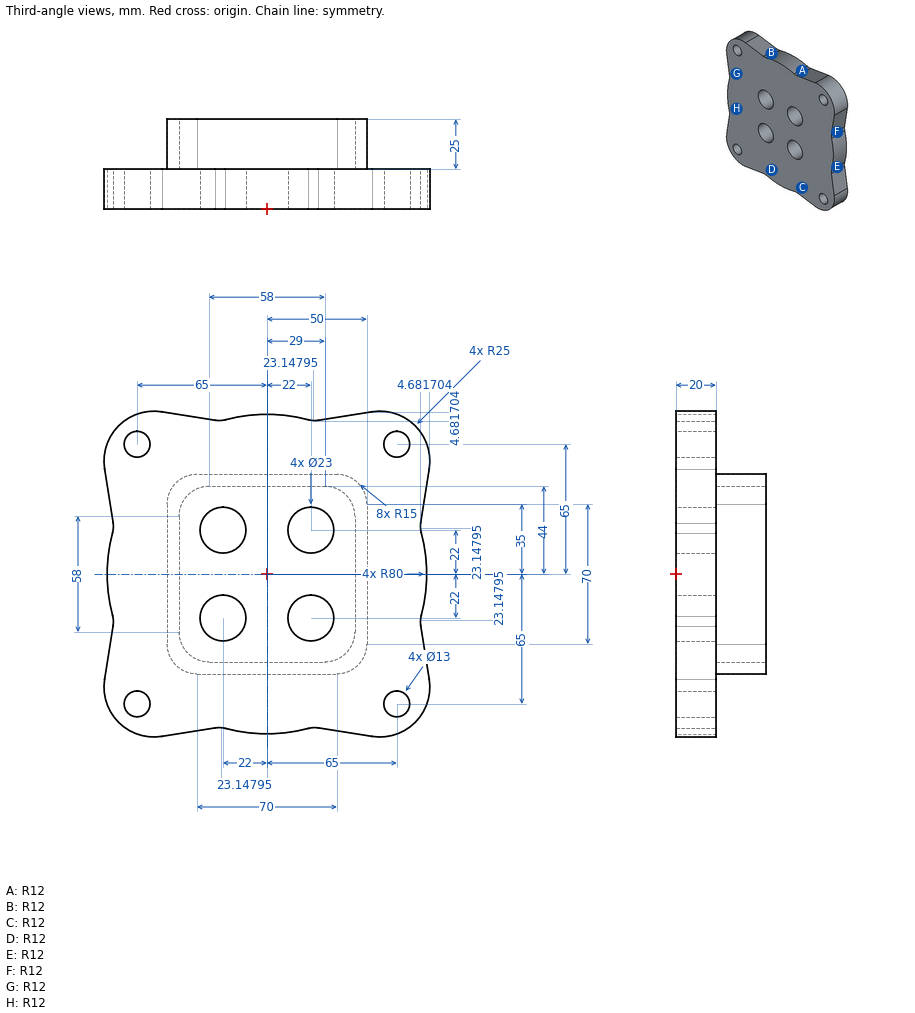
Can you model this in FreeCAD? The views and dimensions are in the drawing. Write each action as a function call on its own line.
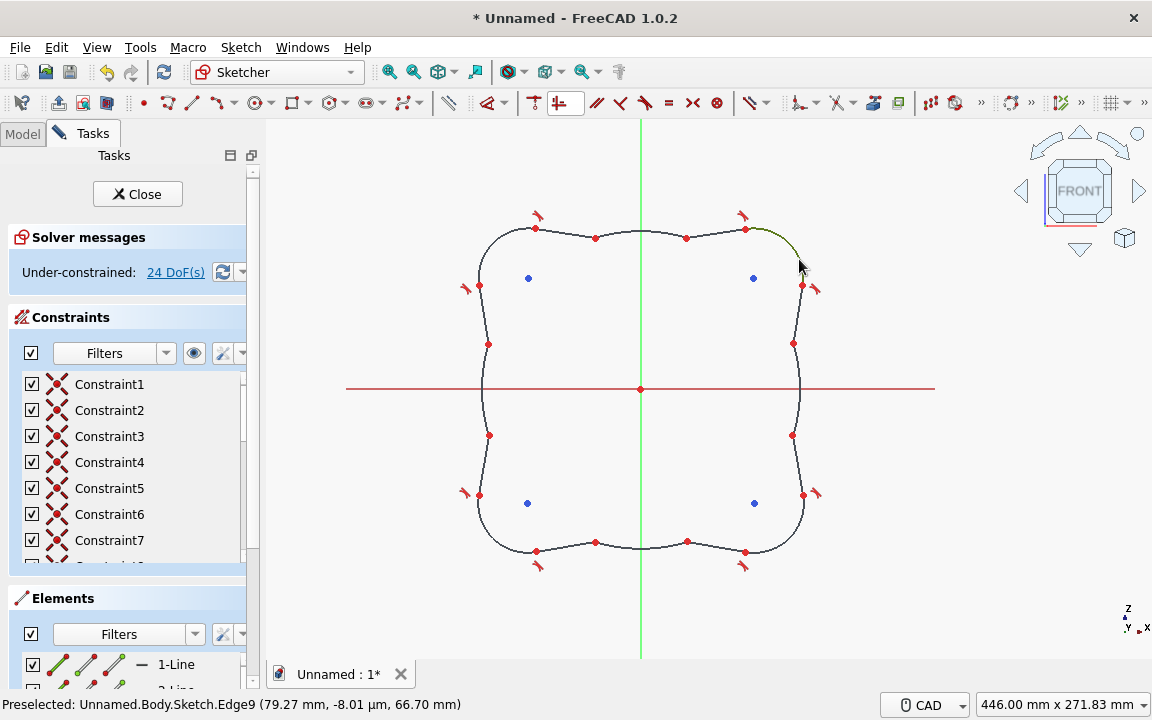
click(774, 549)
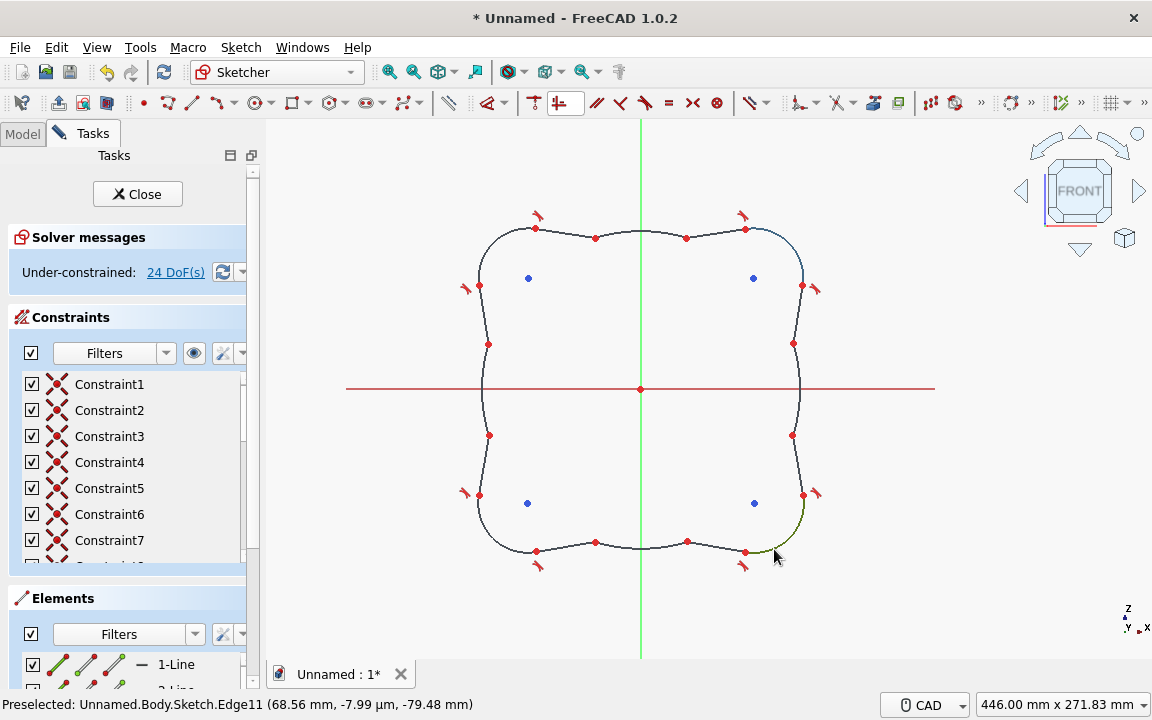
click(482, 523)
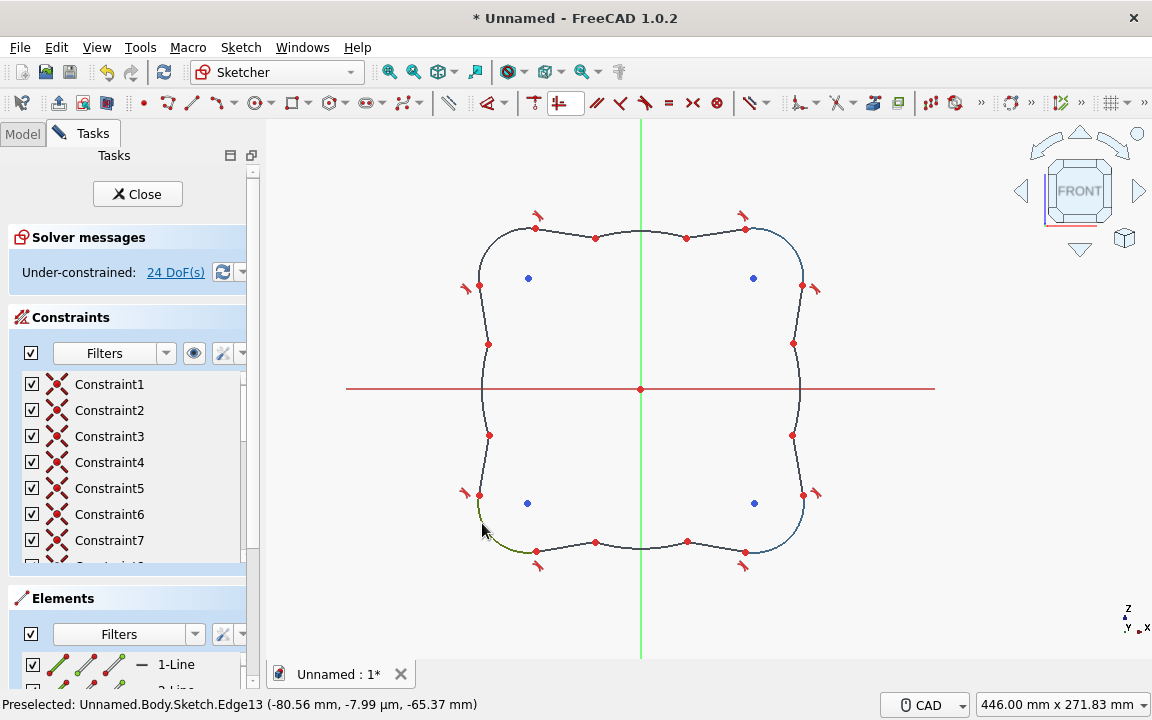
click(509, 233)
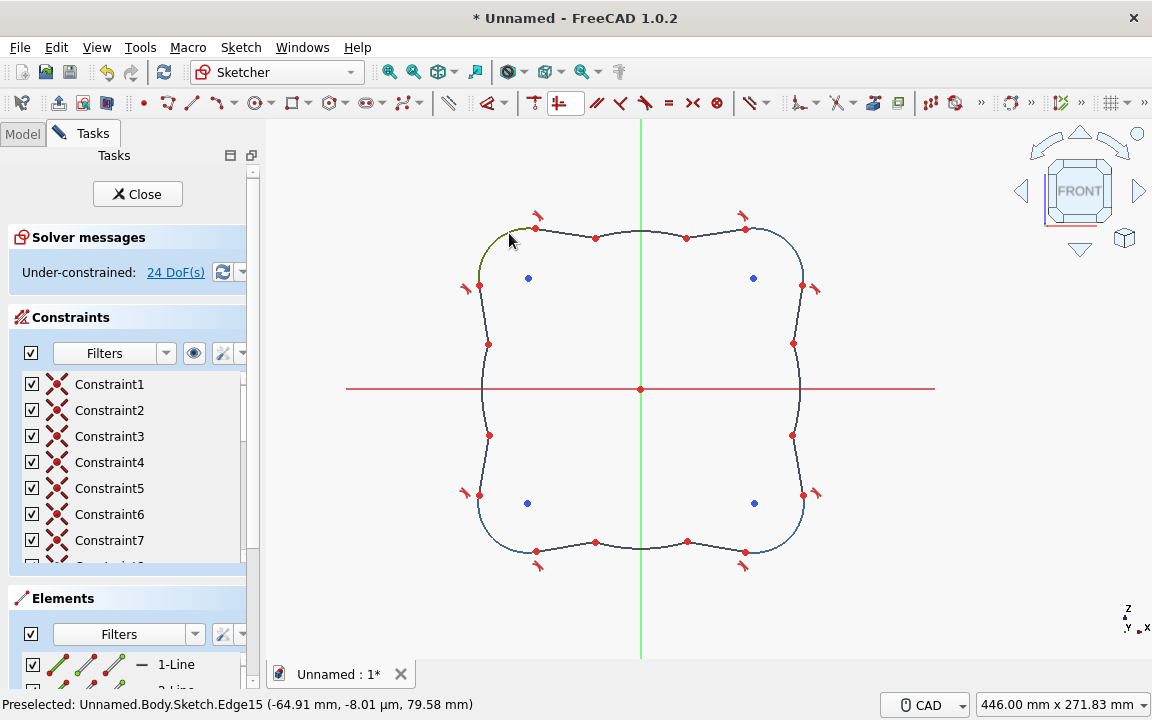
click(670, 104)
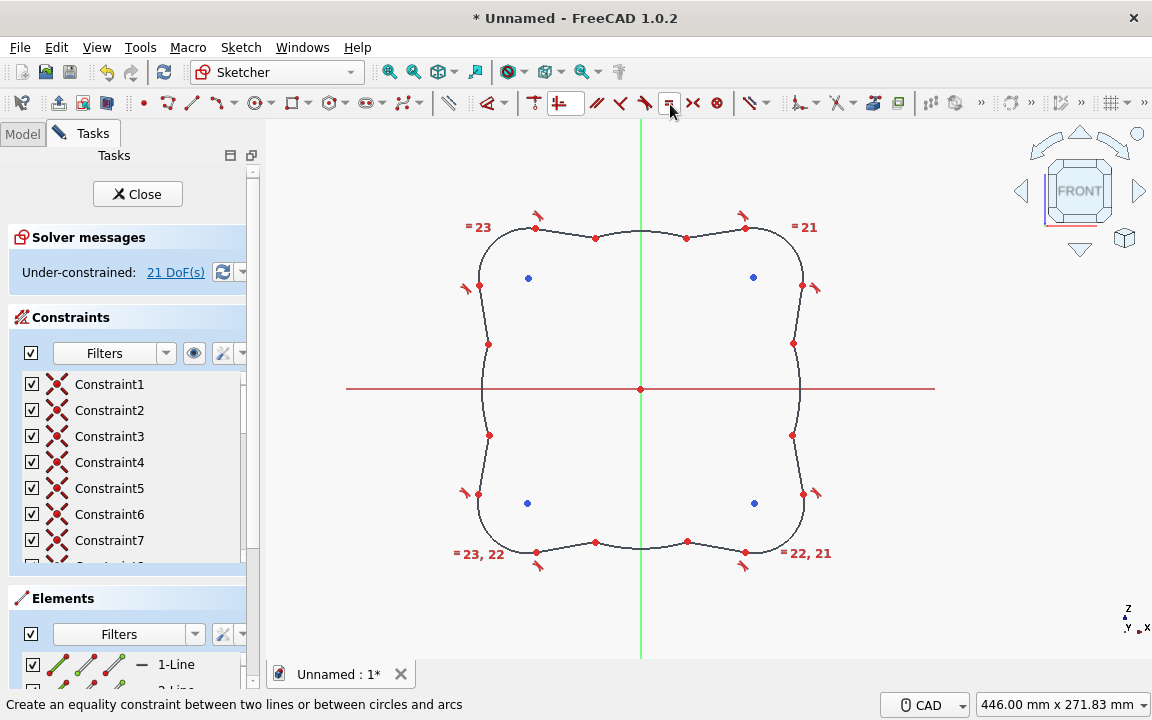
click(799, 409)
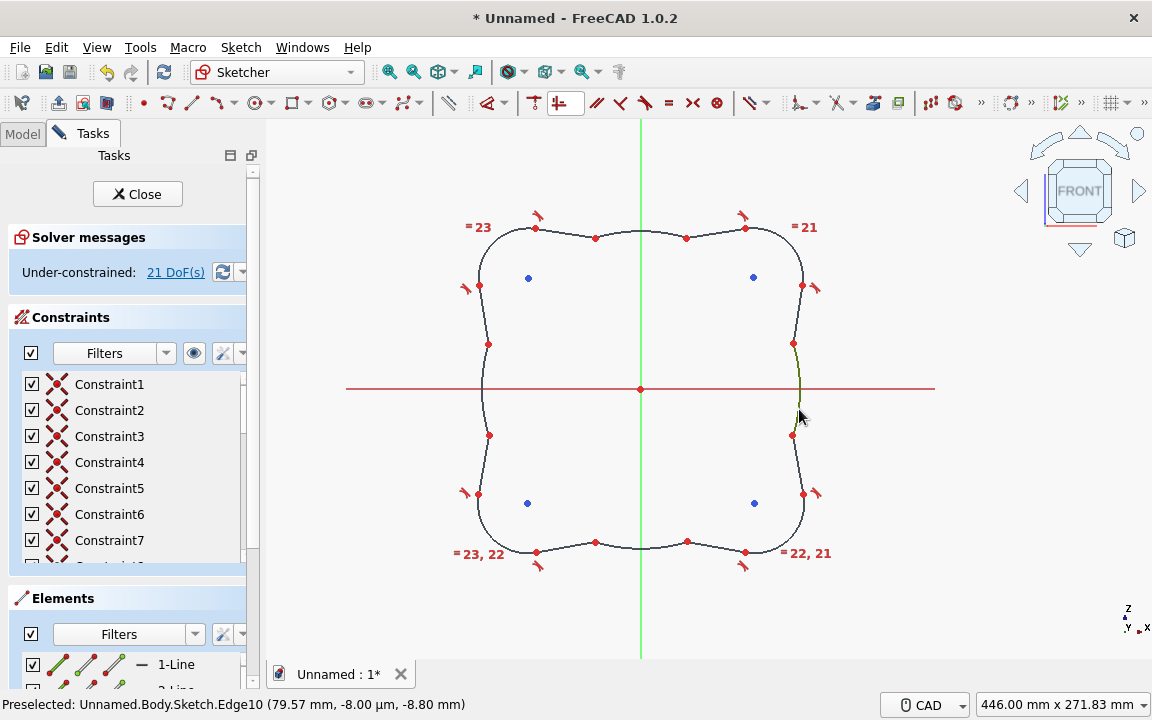
click(622, 548)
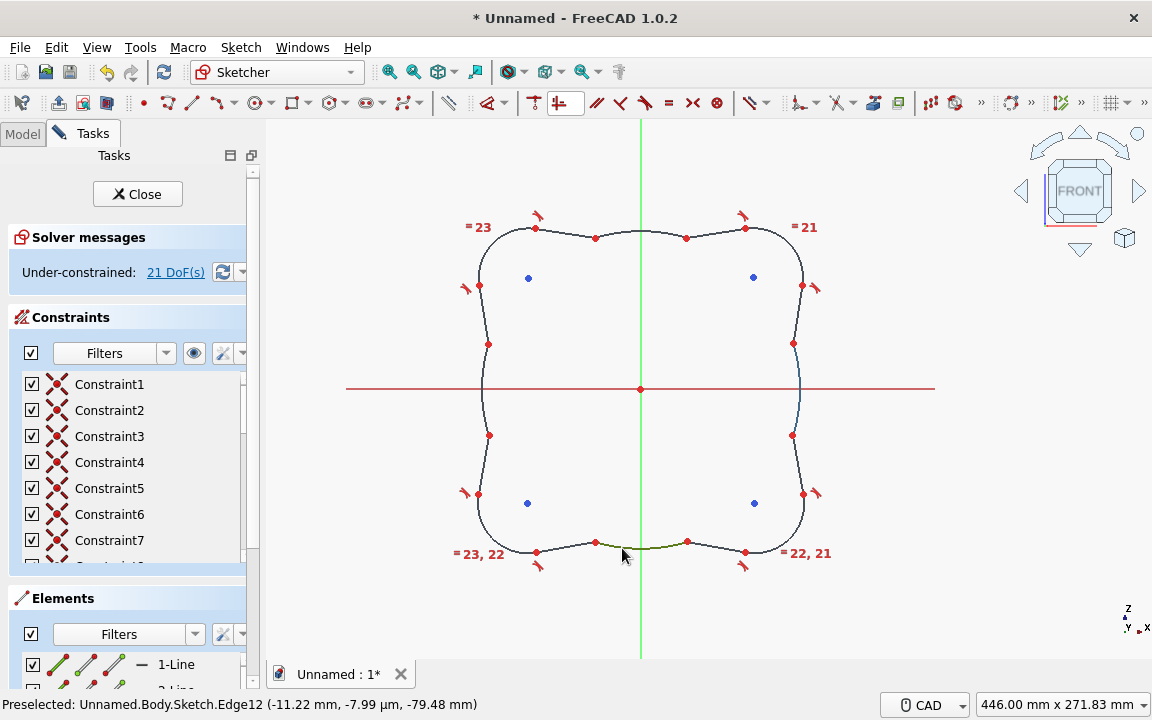
click(483, 371)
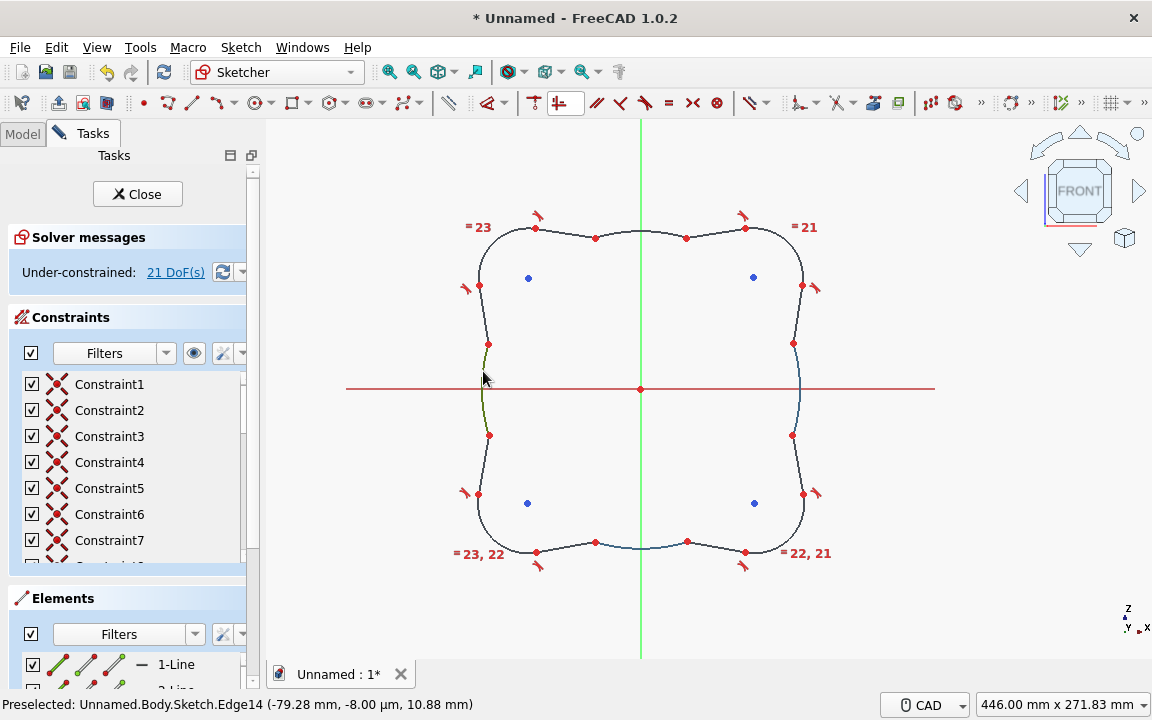
click(660, 232)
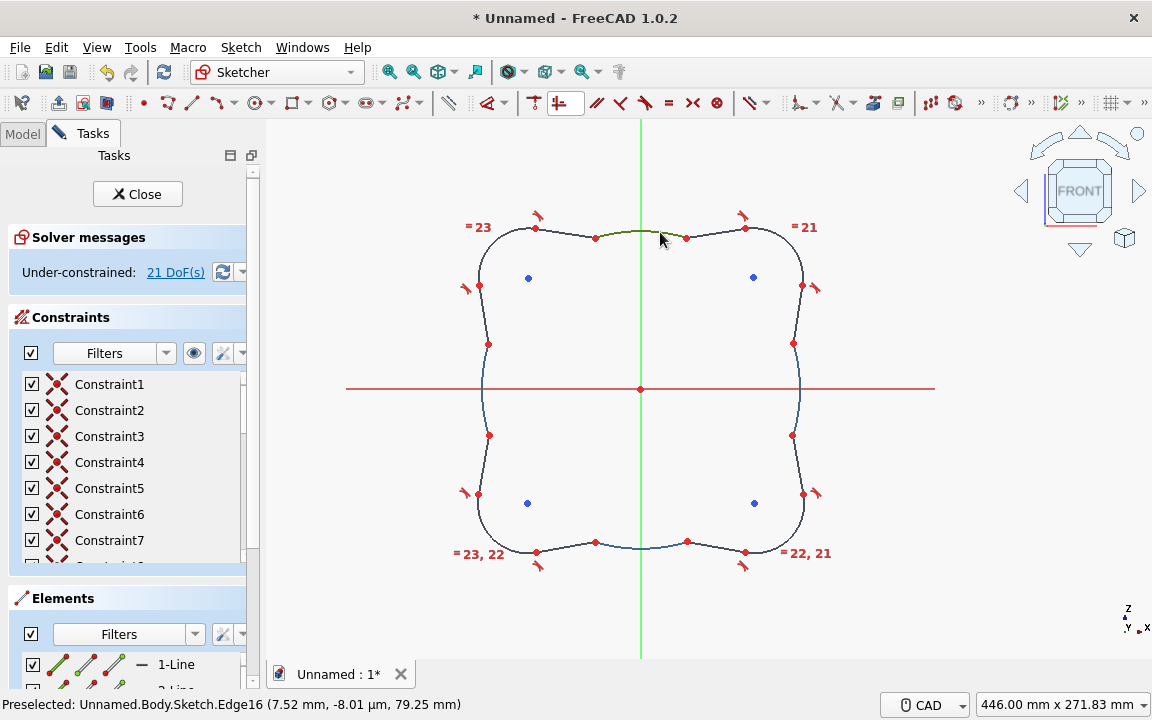
click(670, 104)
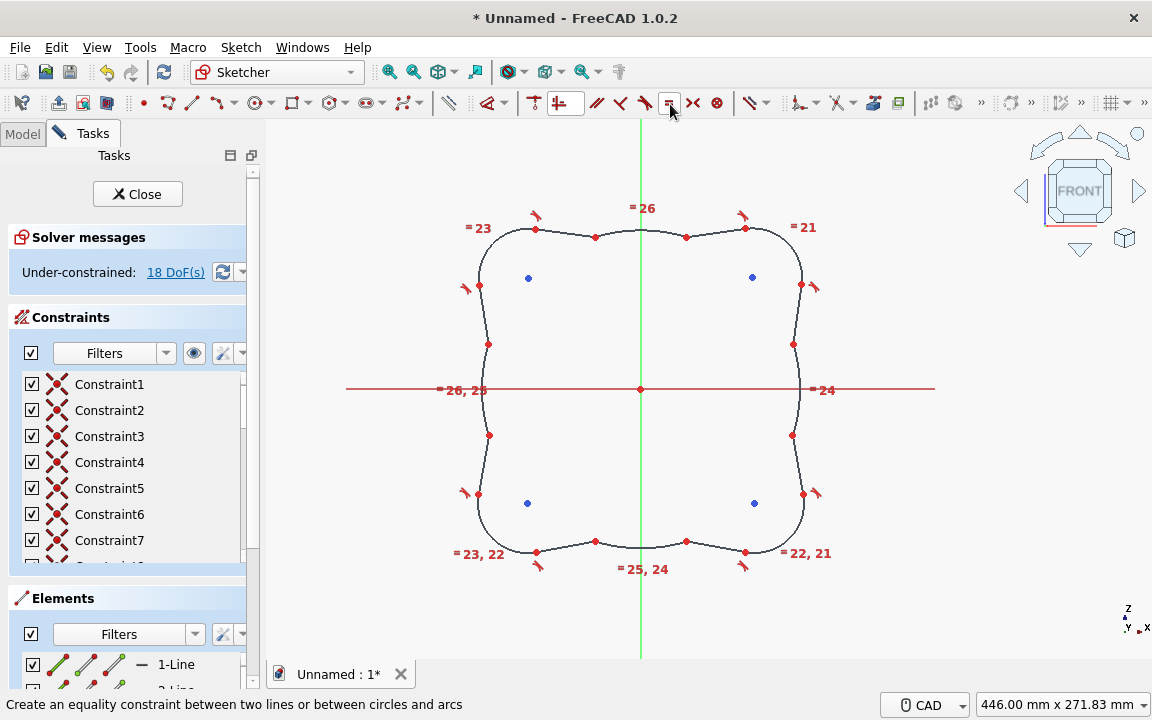
click(753, 278)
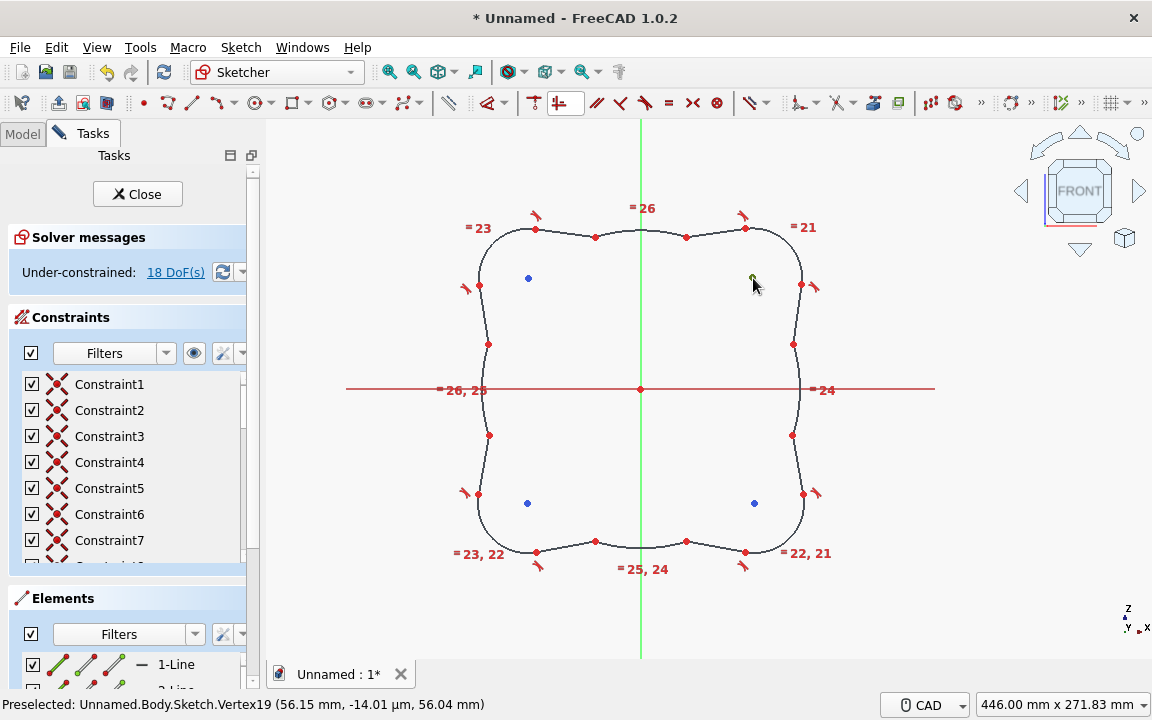
click(754, 503)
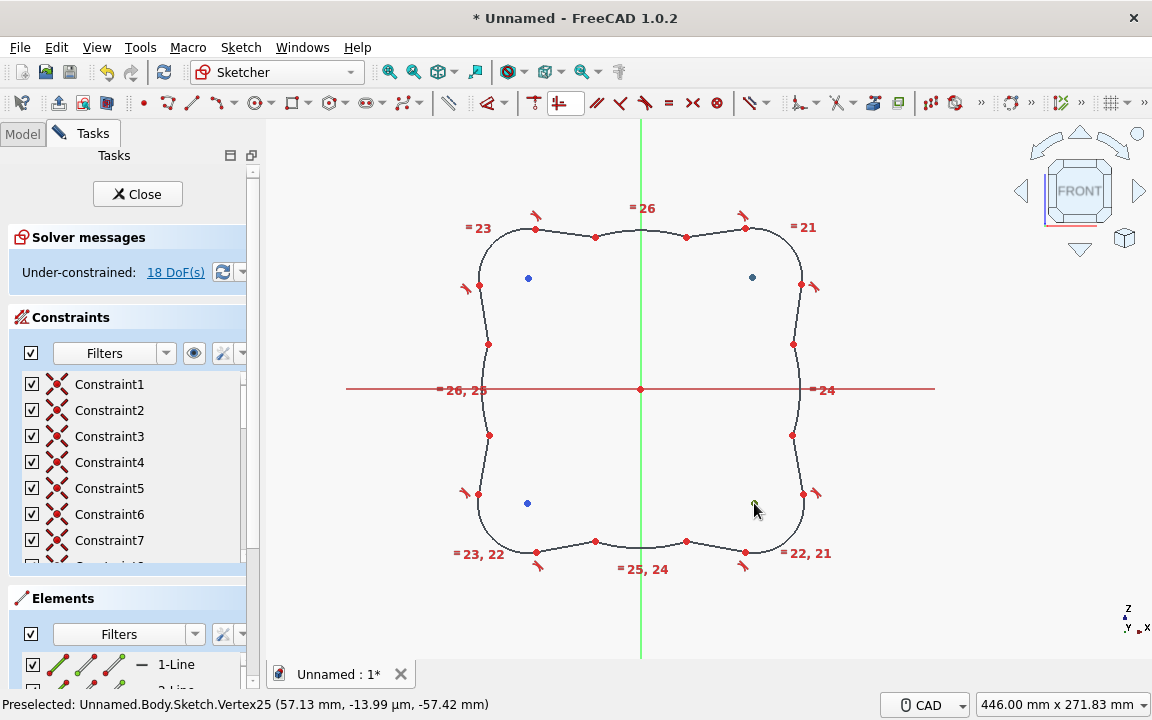
click(344, 389)